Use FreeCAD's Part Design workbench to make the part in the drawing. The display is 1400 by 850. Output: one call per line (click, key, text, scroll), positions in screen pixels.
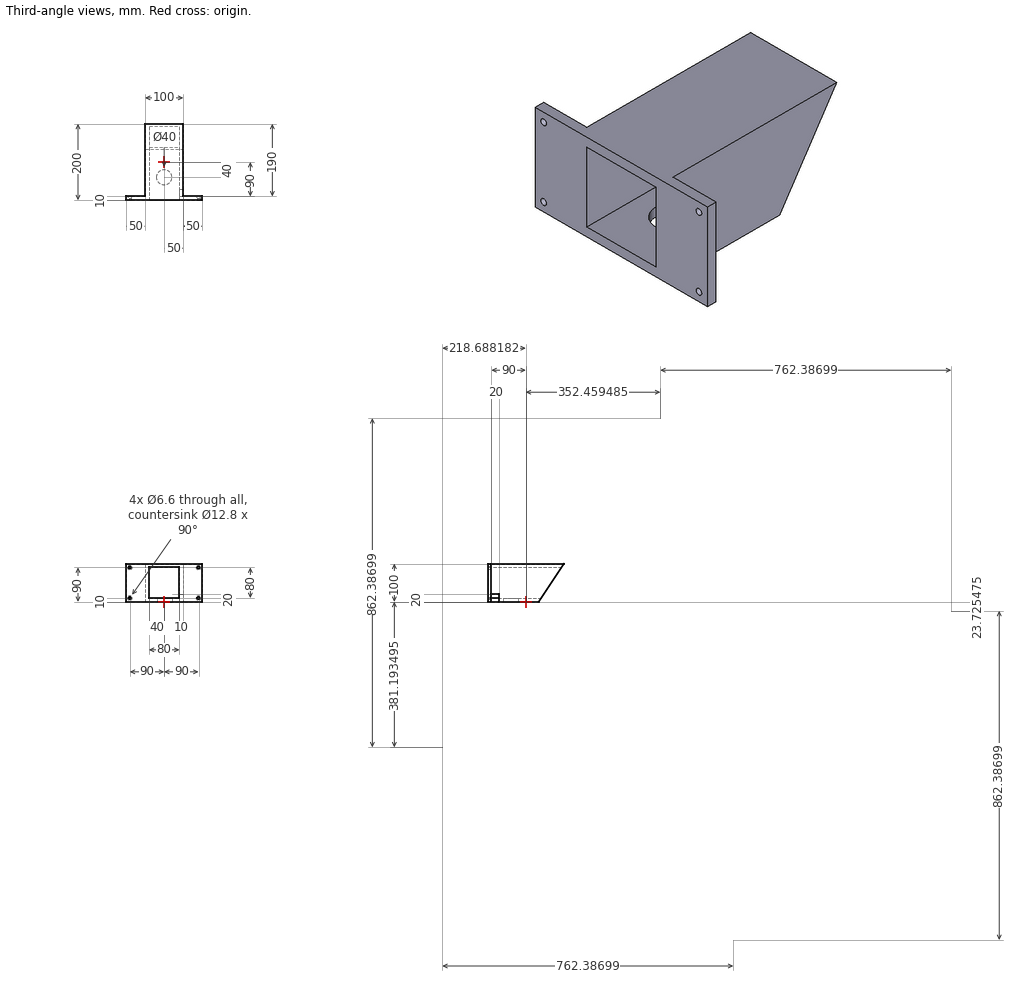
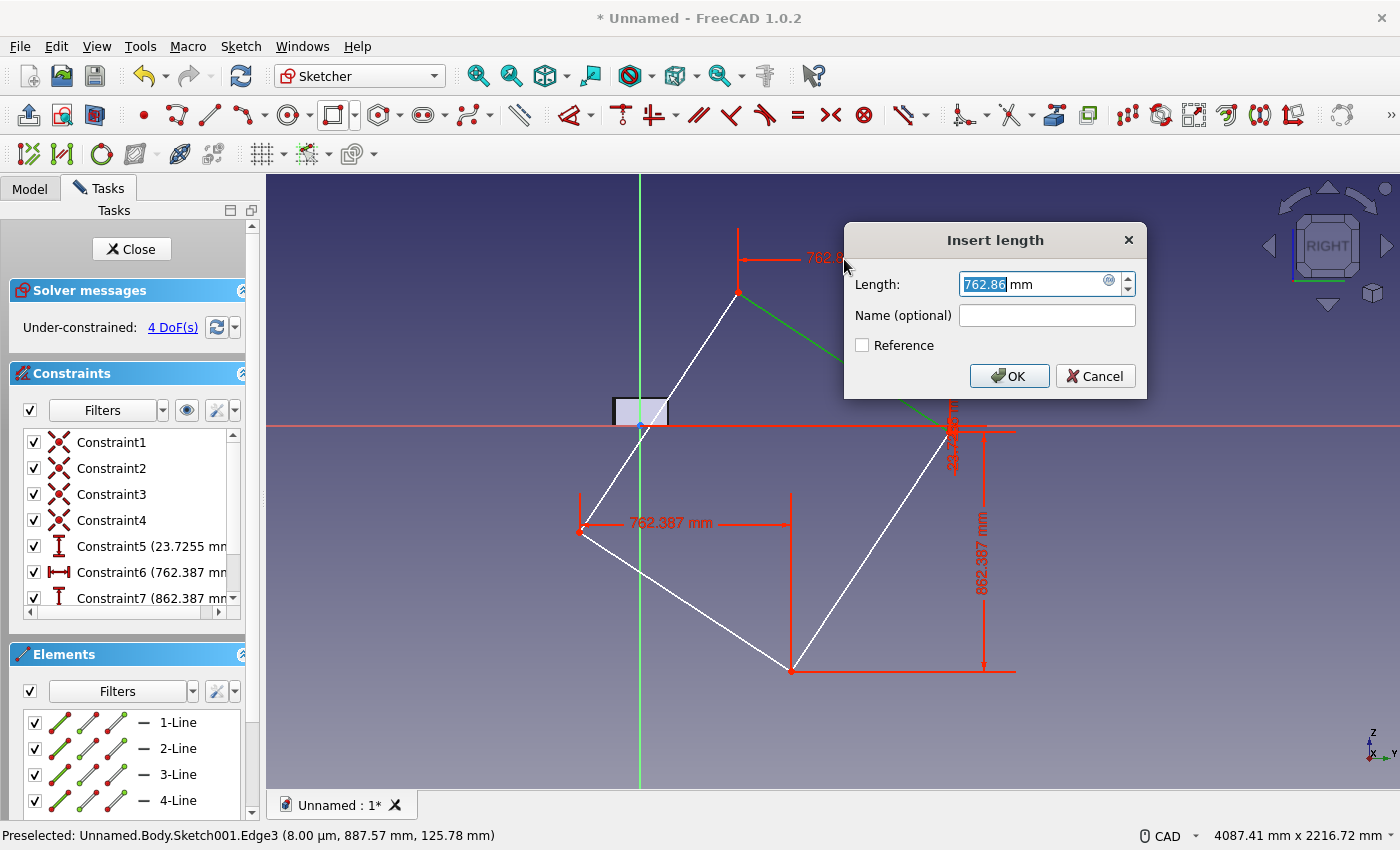
text(762.38699)
key(Return)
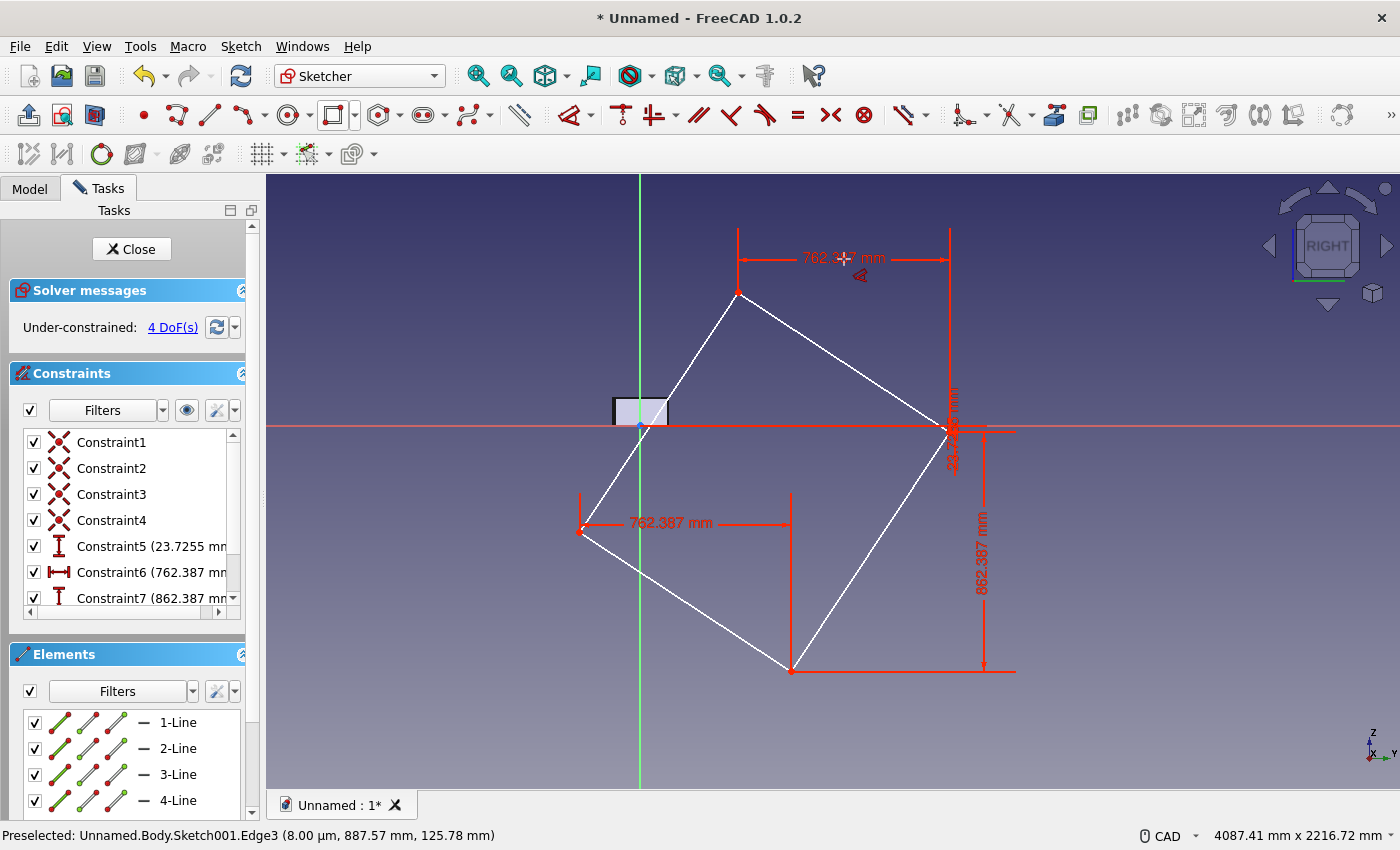
click(691, 365)
click(546, 413)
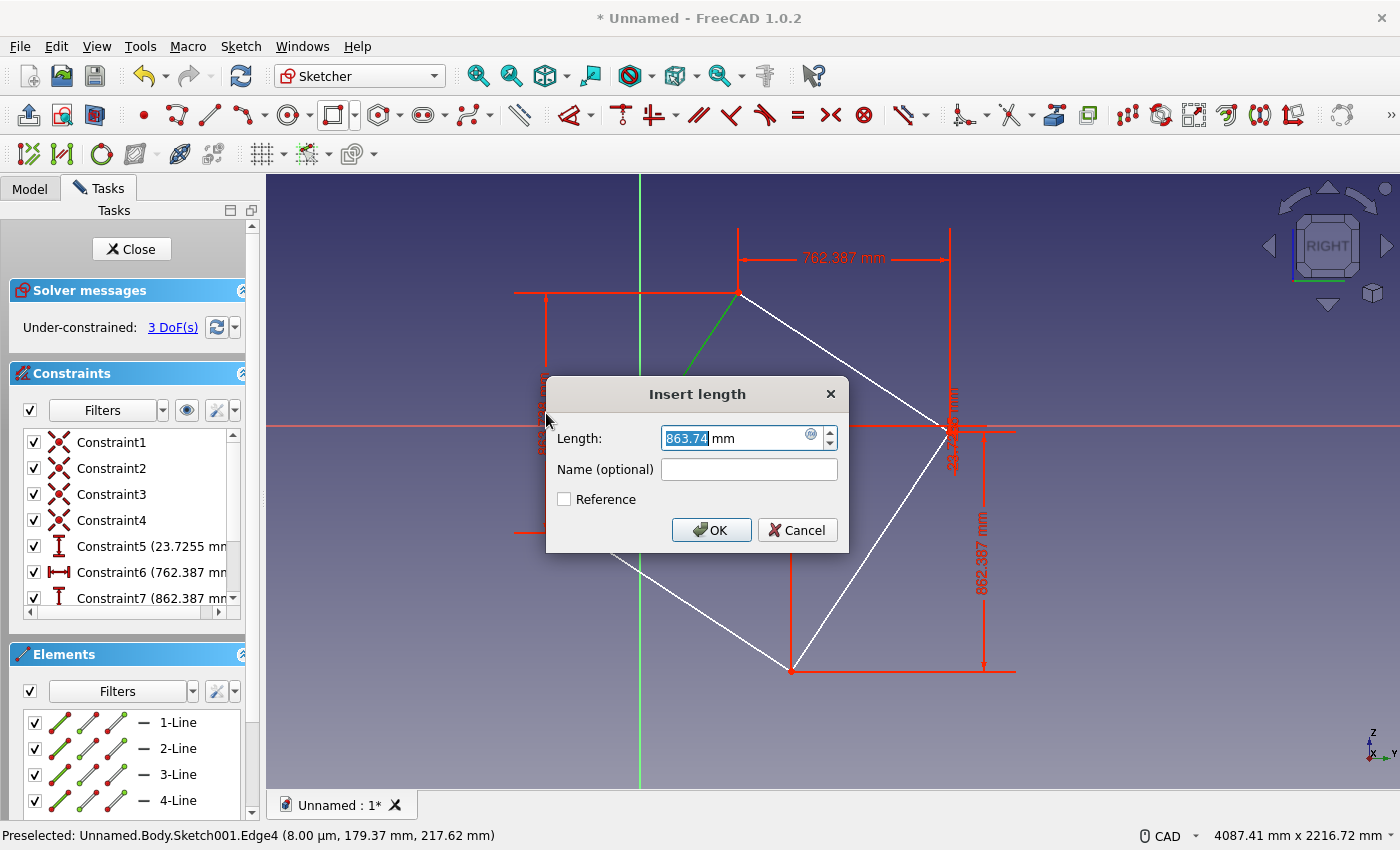
text(862.38699)
key(Return)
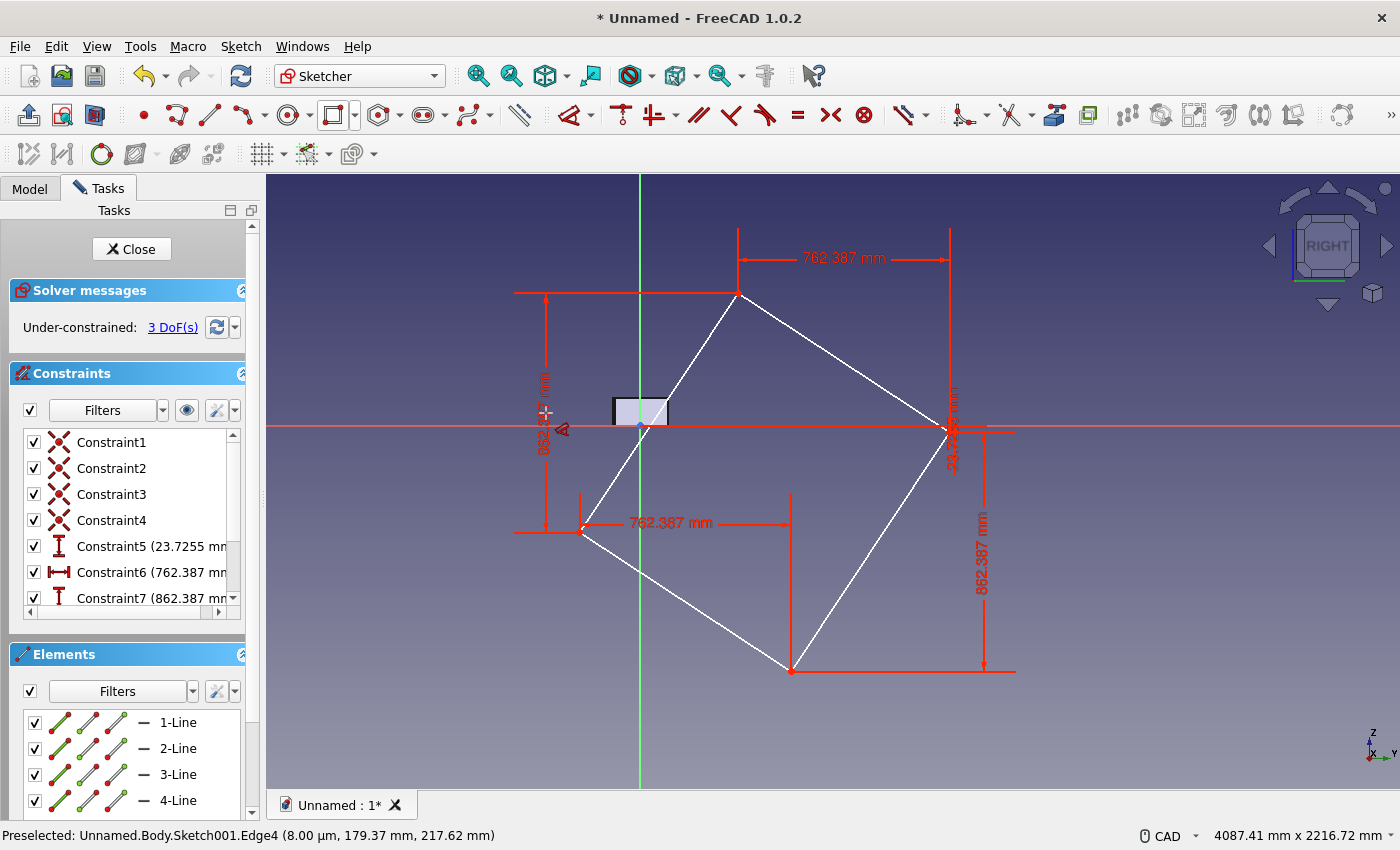
click(580, 533)
click(610, 392)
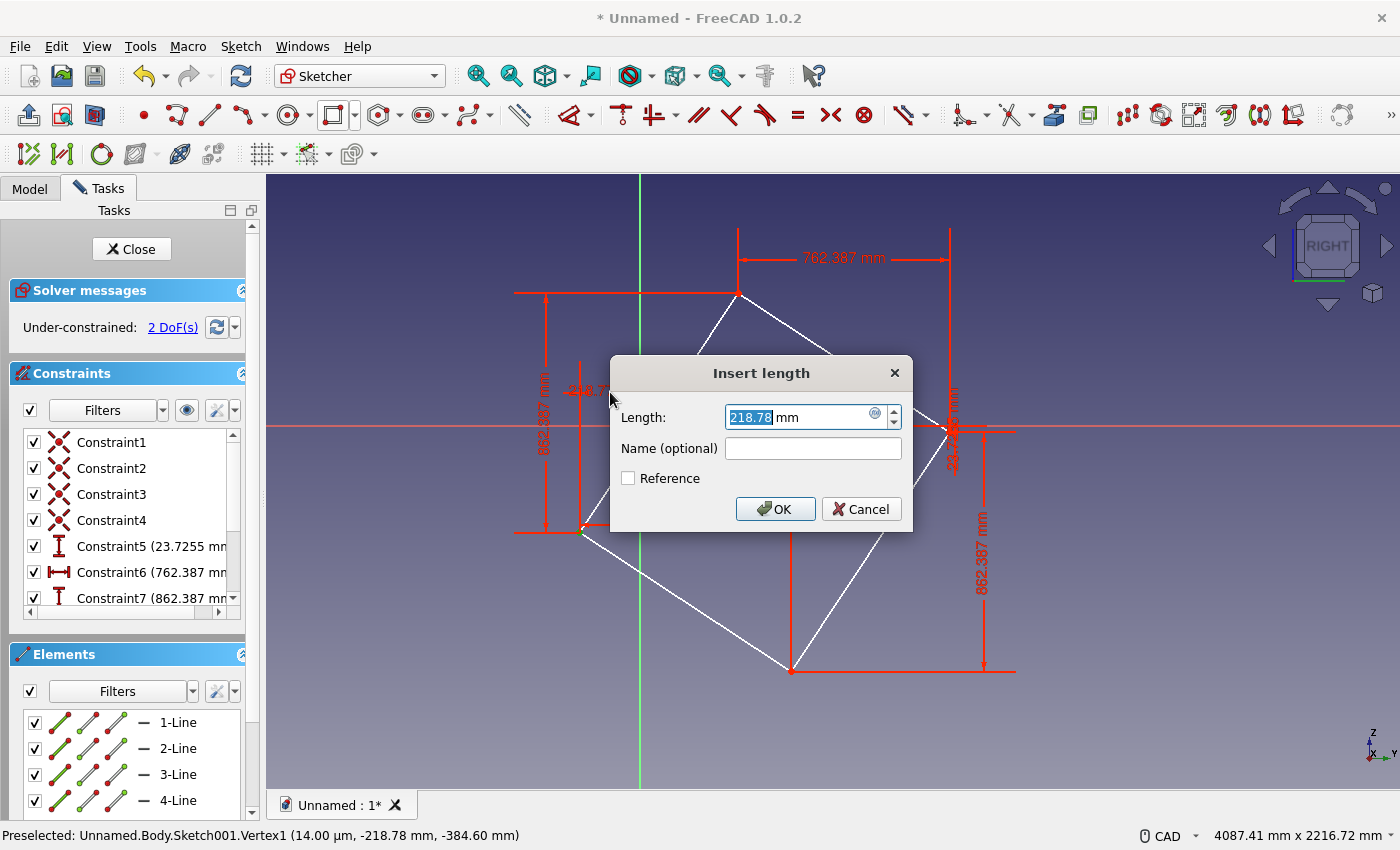
text(218.688182)
key(Return)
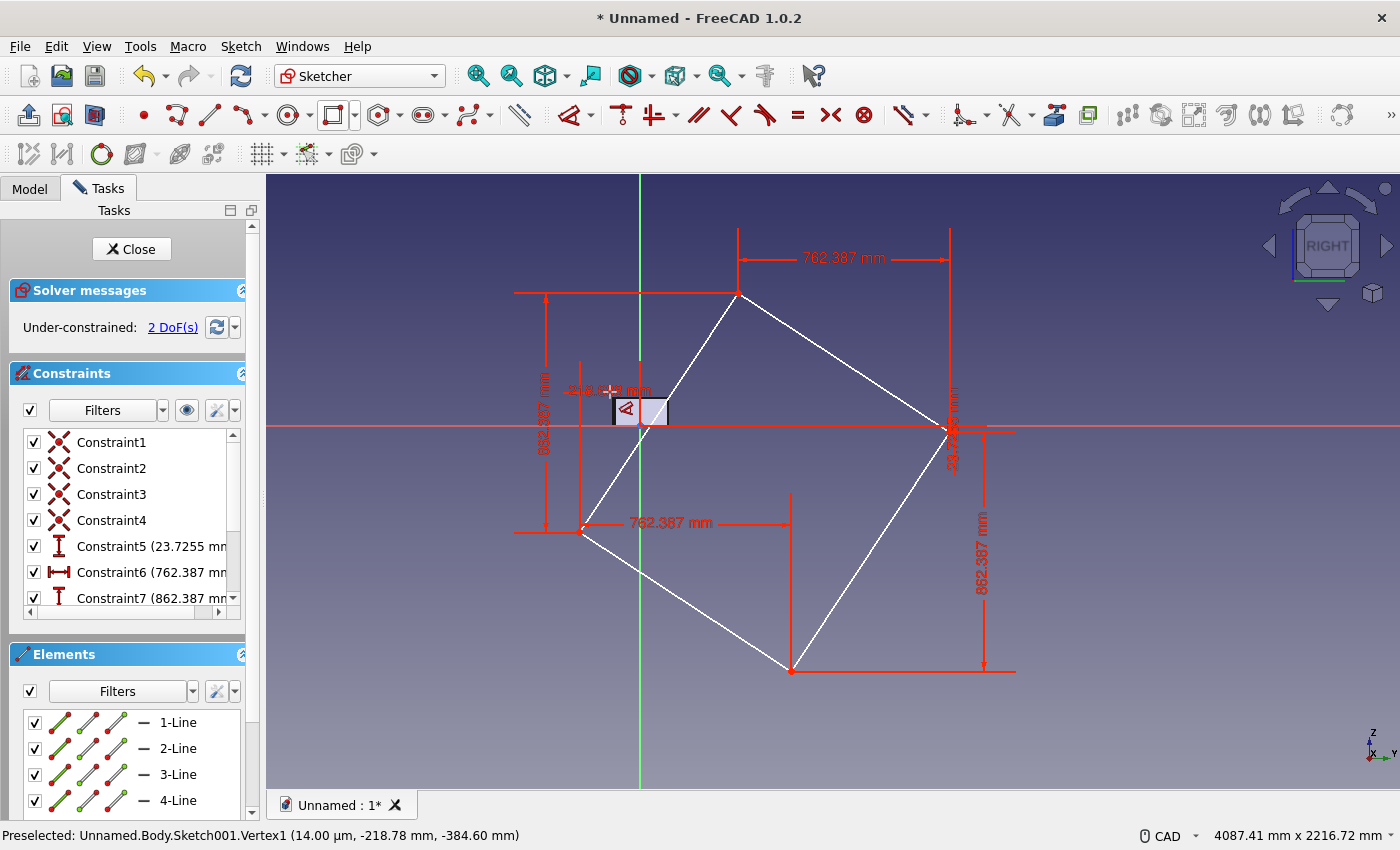
click(580, 533)
click(546, 479)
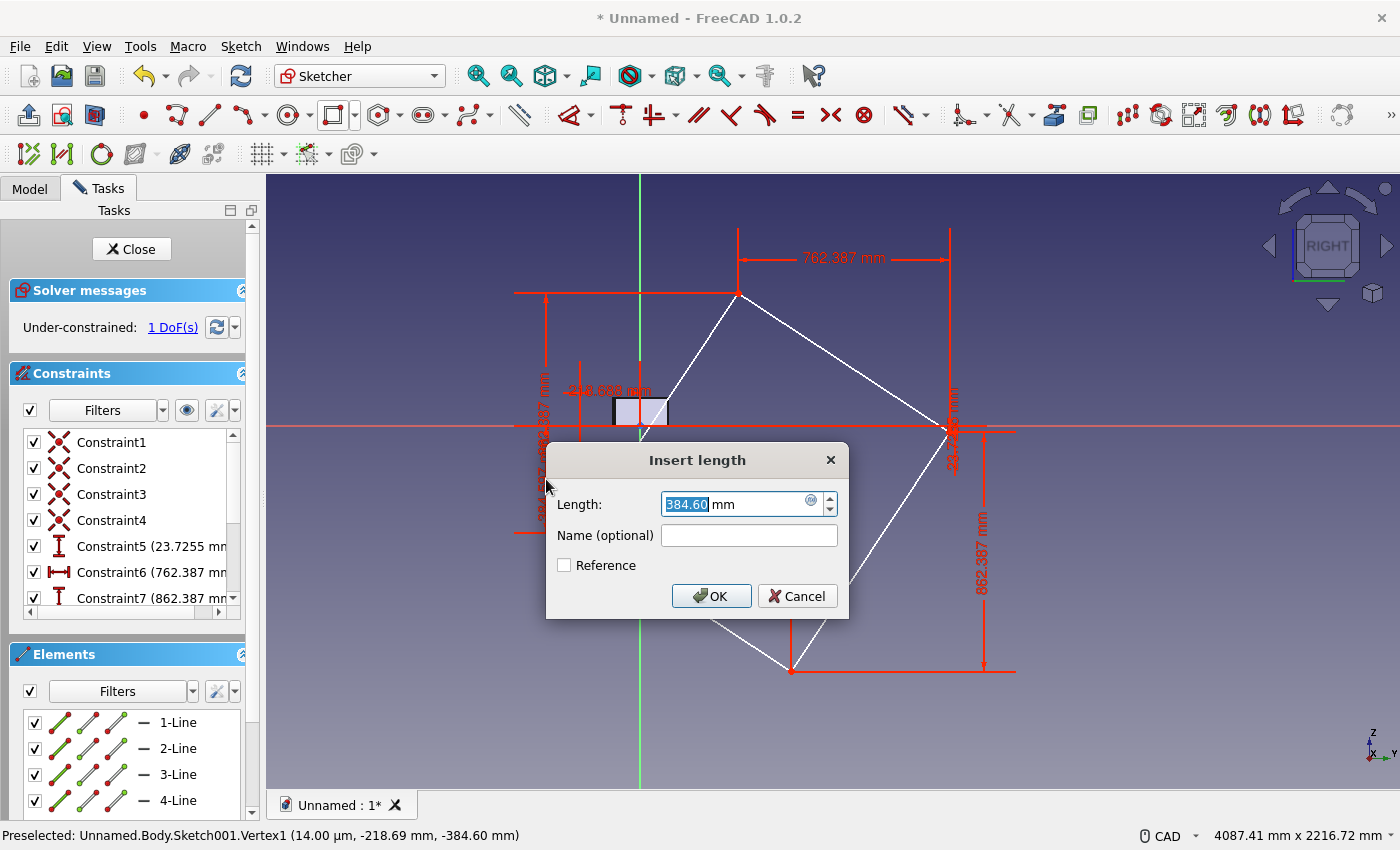
text(381.193495)
key(Return)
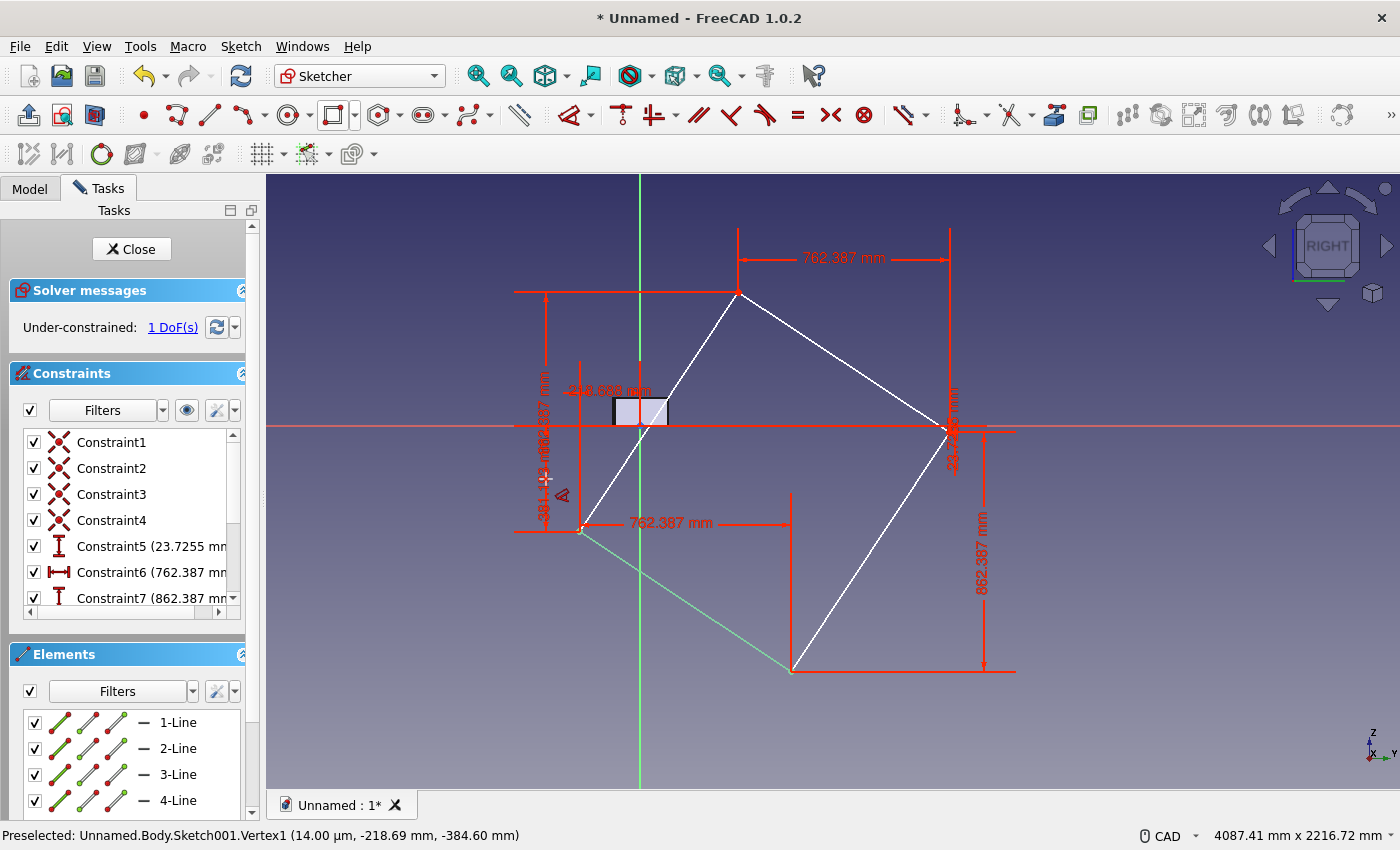
click(738, 292)
click(689, 258)